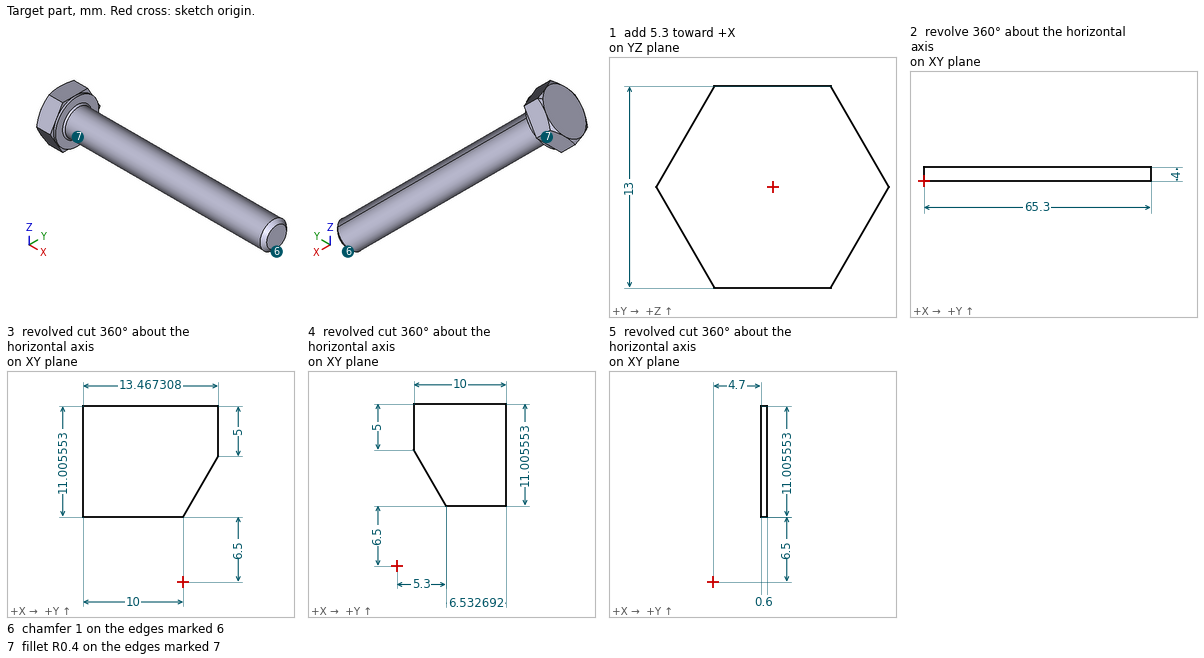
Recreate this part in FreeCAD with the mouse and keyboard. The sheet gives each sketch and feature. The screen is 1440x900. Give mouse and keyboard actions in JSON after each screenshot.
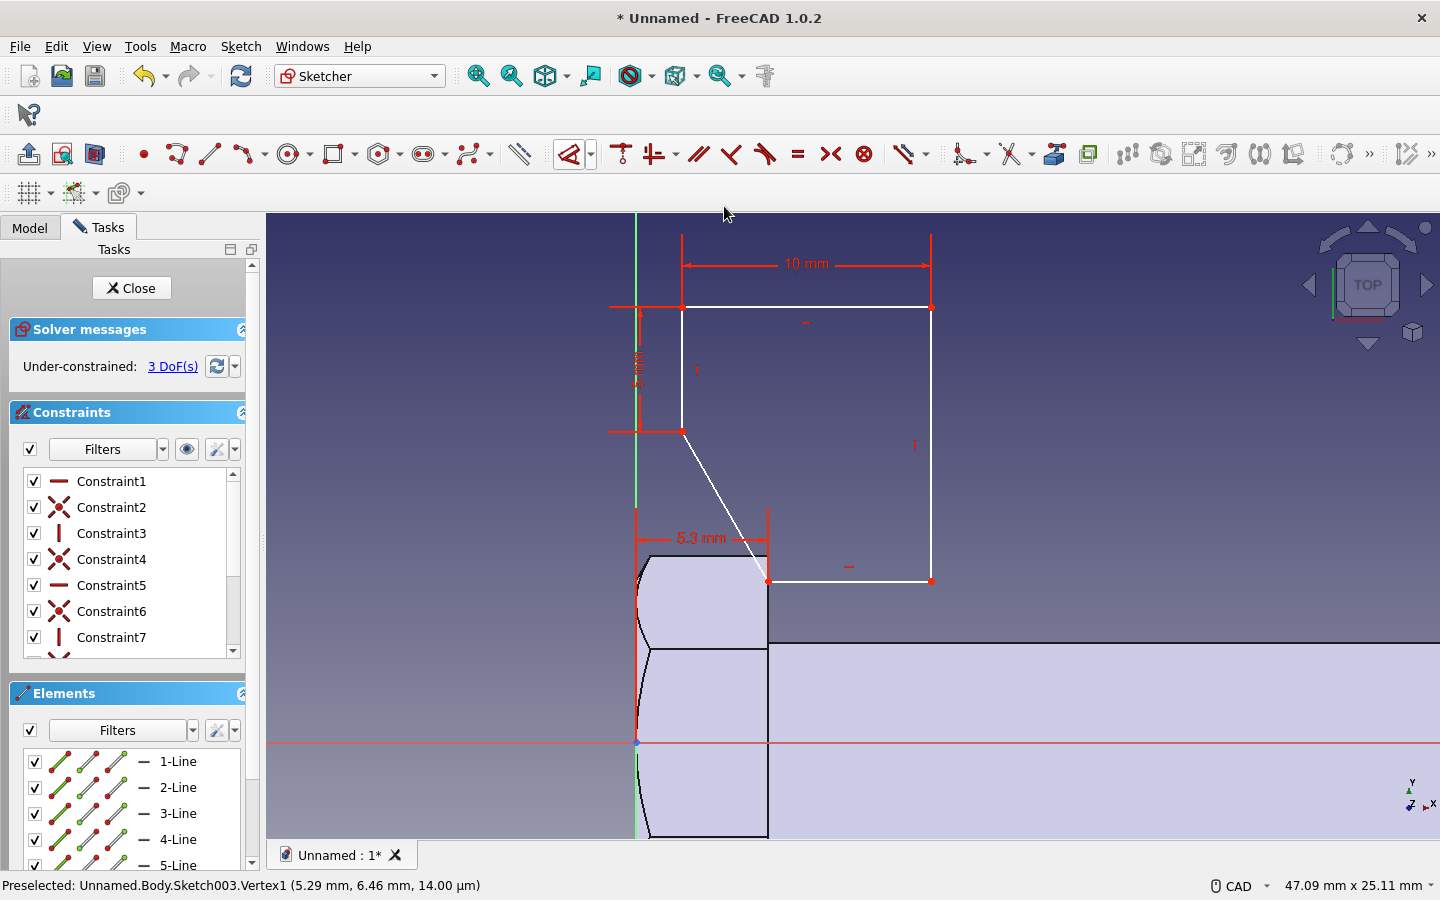
{"action": "left_click", "coordinate": [768, 582]}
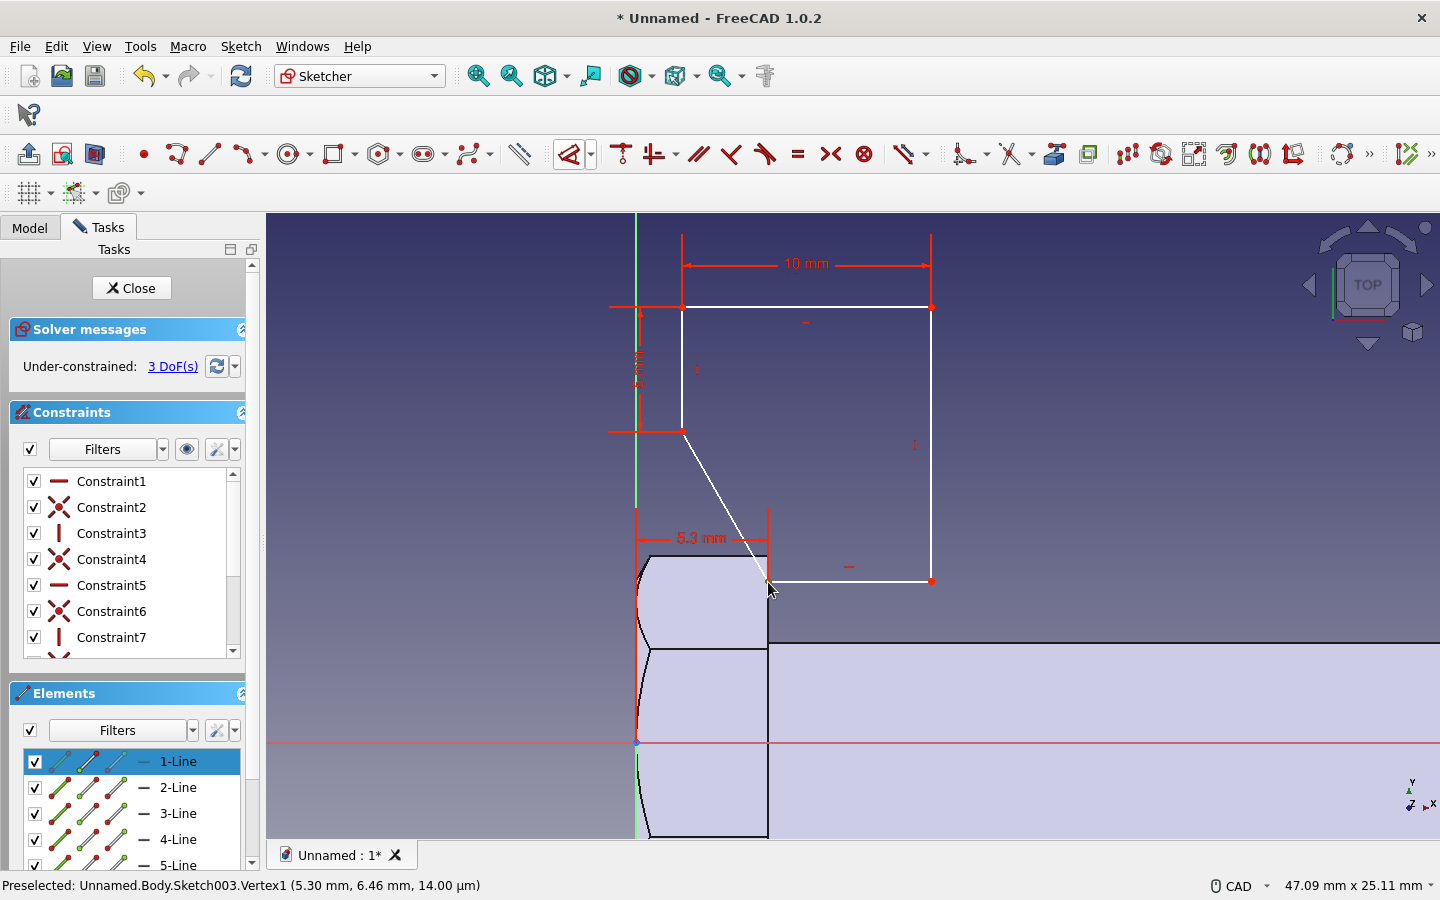
{"action": "key", "text": "i"}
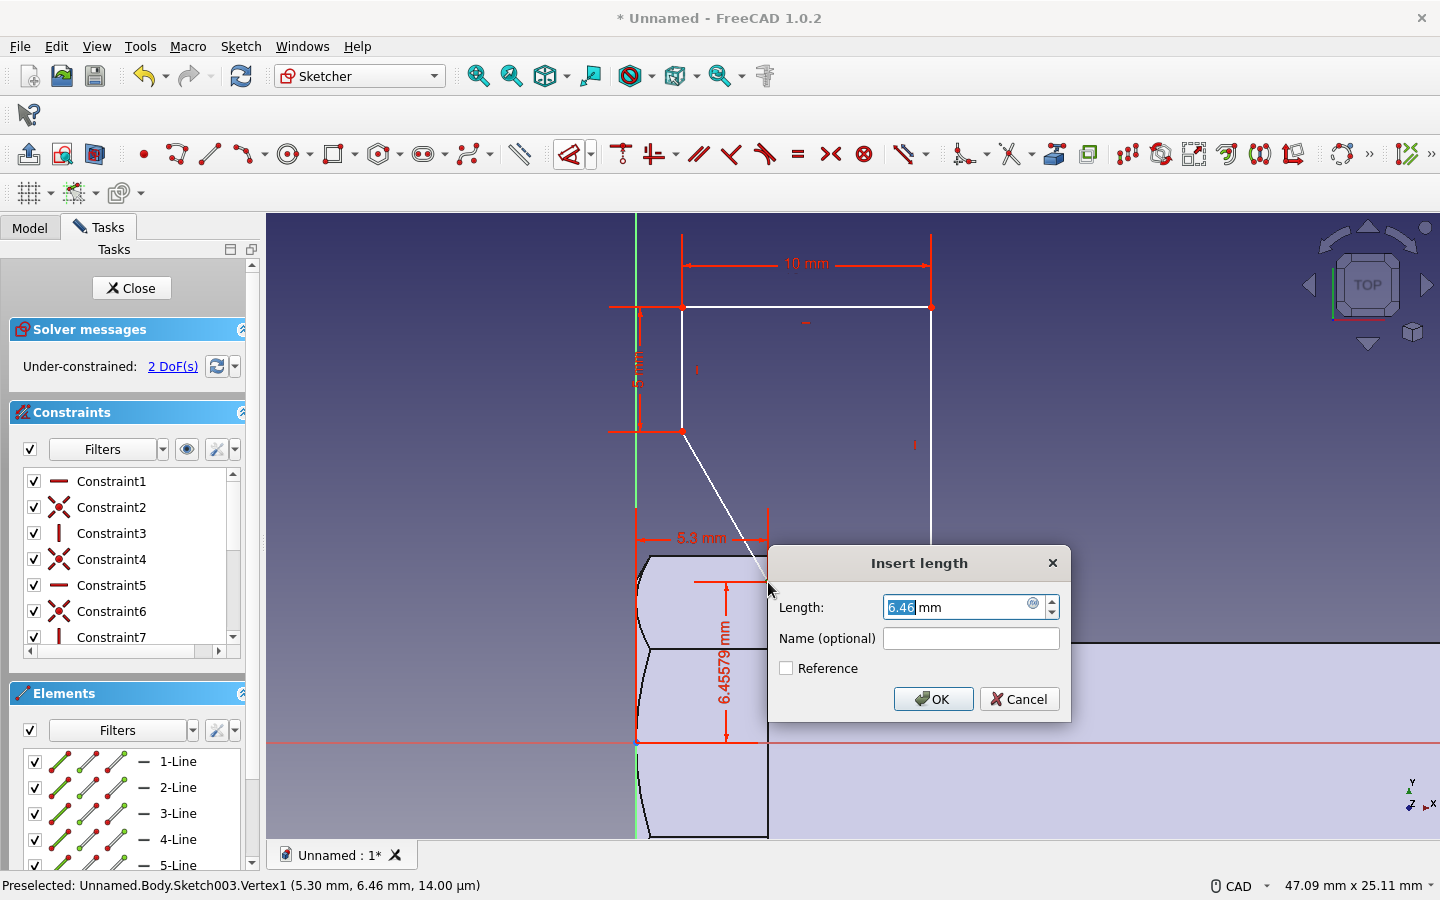
{"action": "type", "text": "6.5"}
{"action": "key", "text": "Return"}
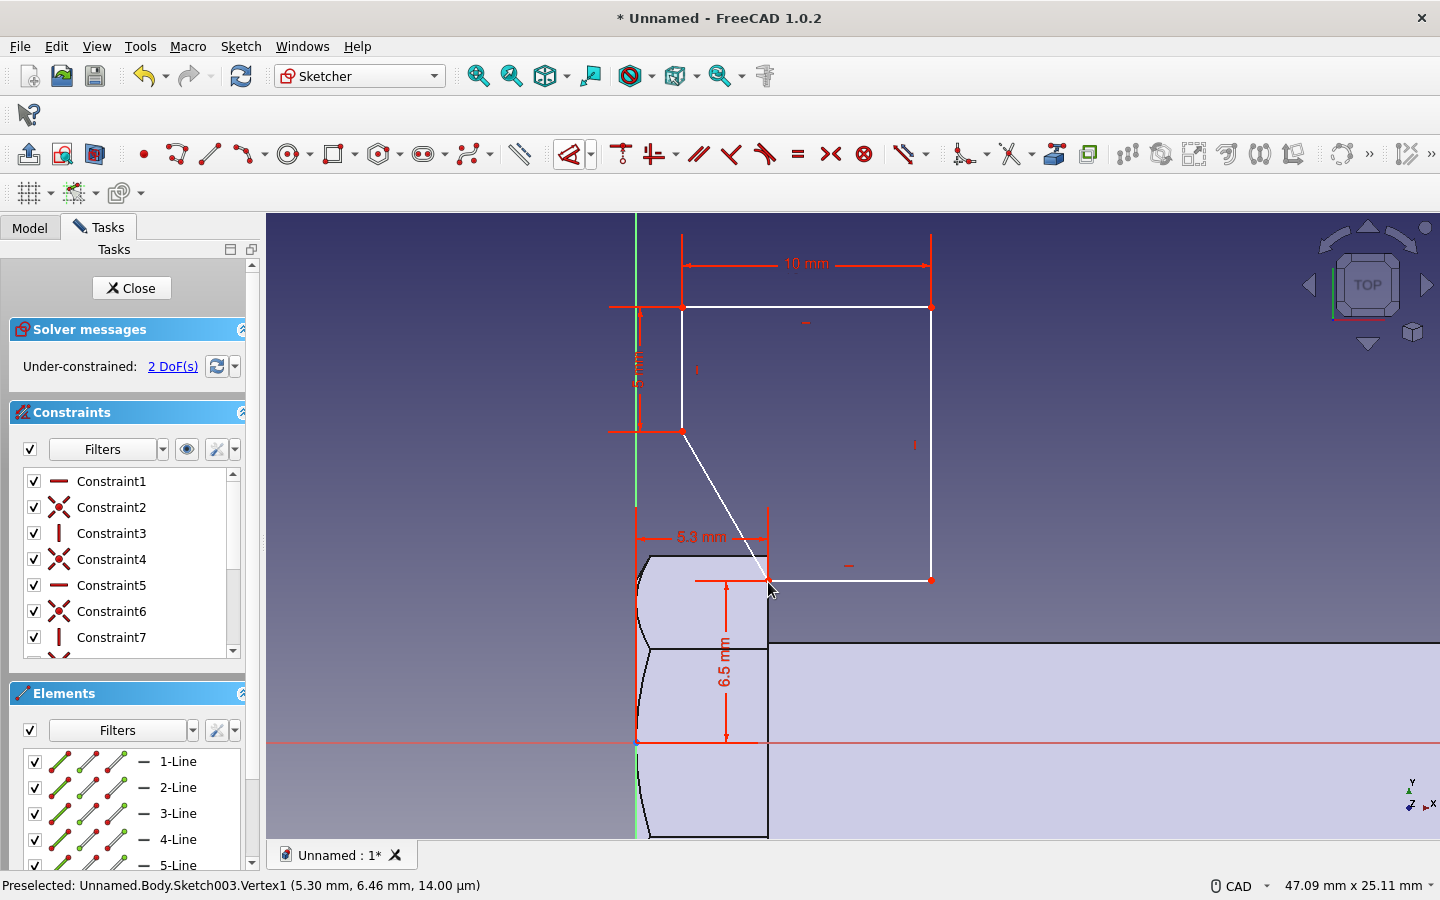
{"action": "left_click", "coordinate": [817, 581]}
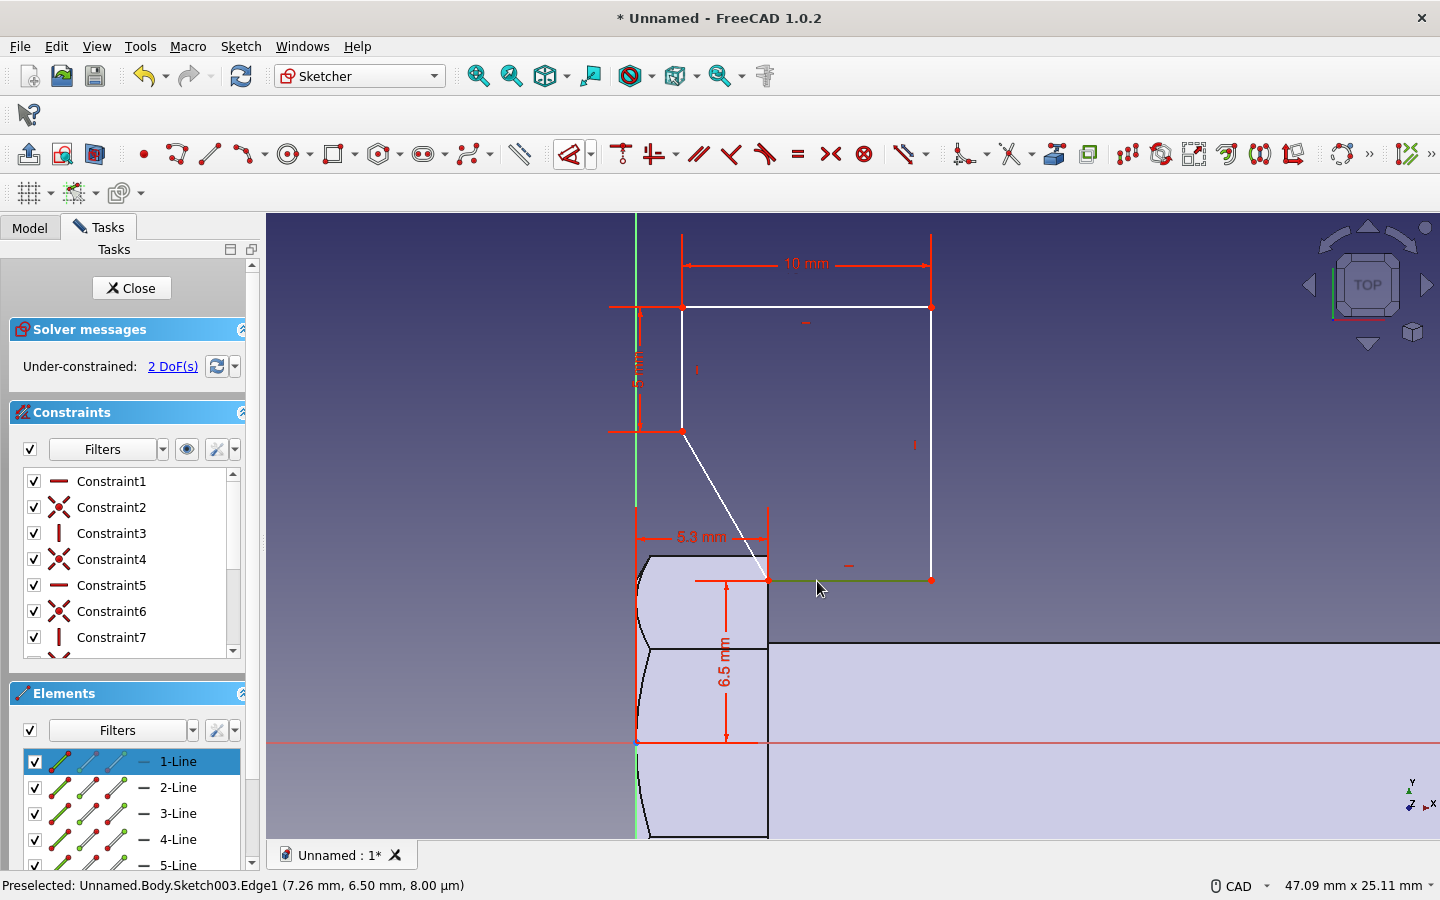
{"action": "key", "text": "l"}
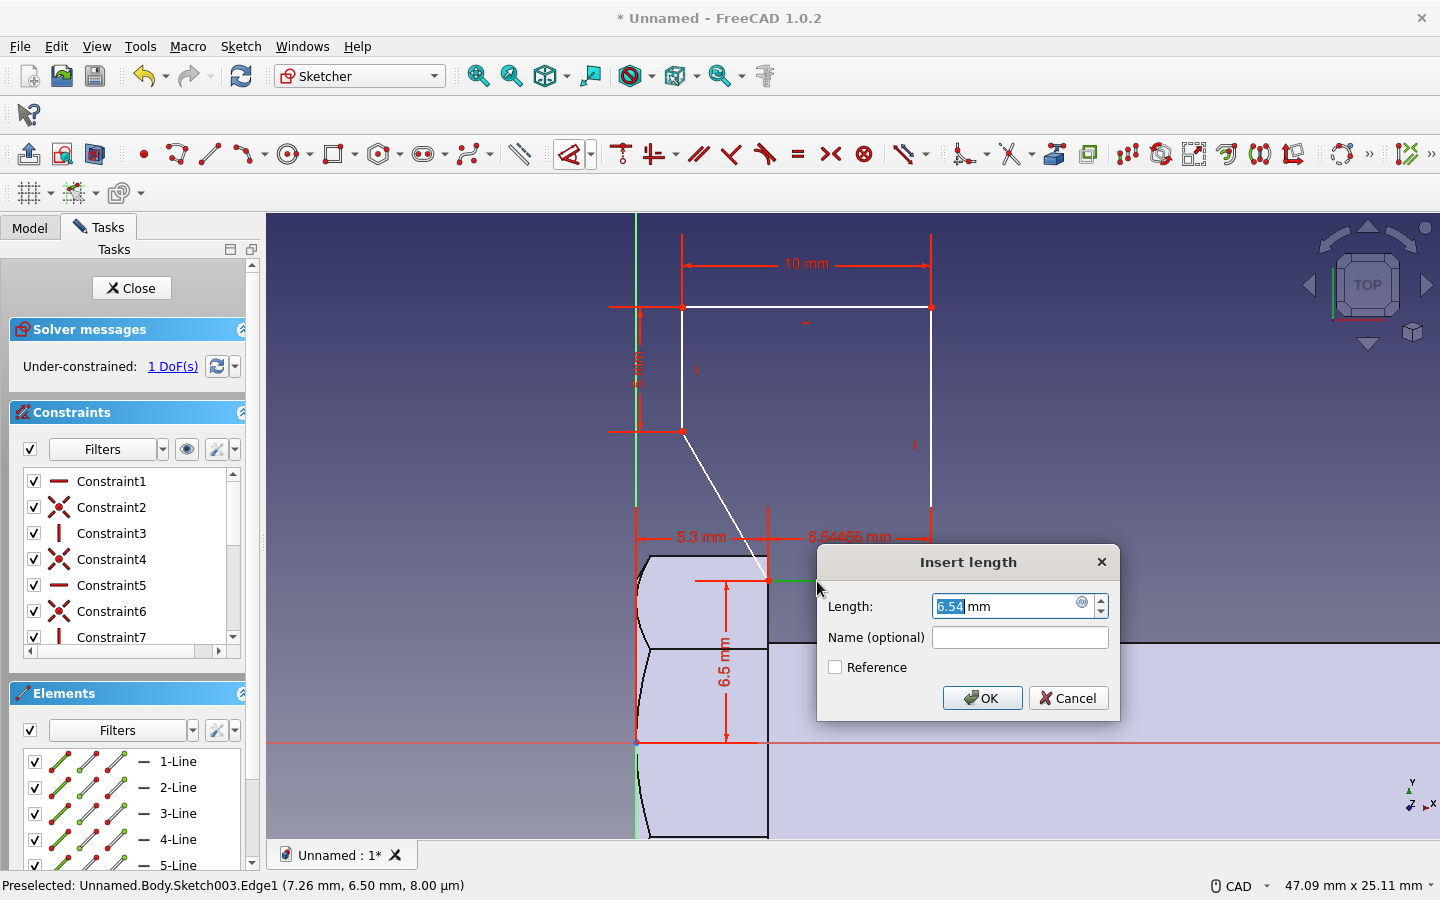
{"action": "type", "text": "6.532692"}
{"action": "key", "text": "Return"}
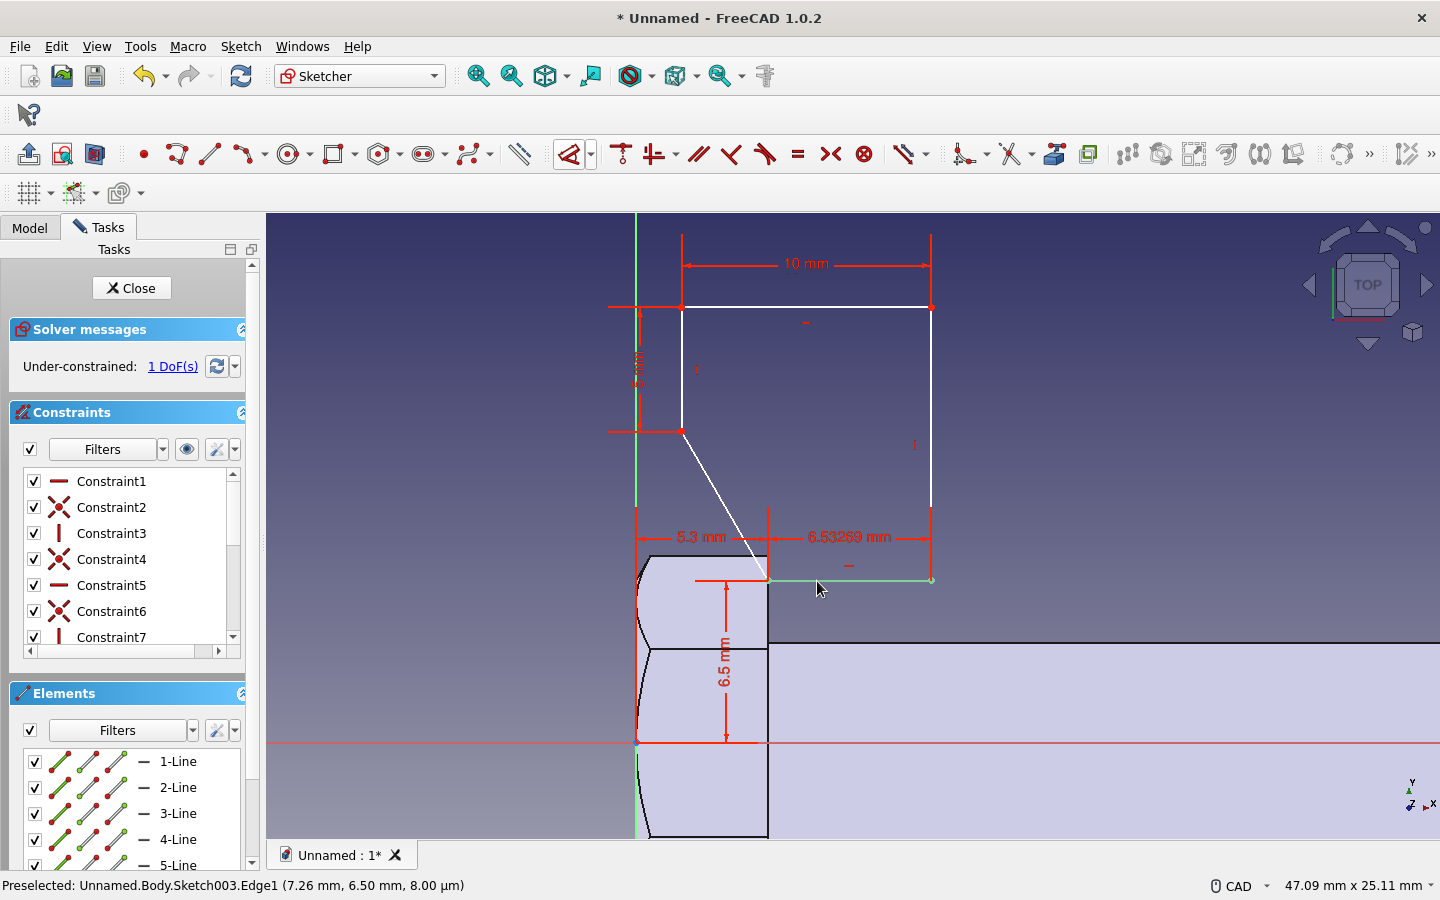
{"action": "left_click", "coordinate": [931, 499]}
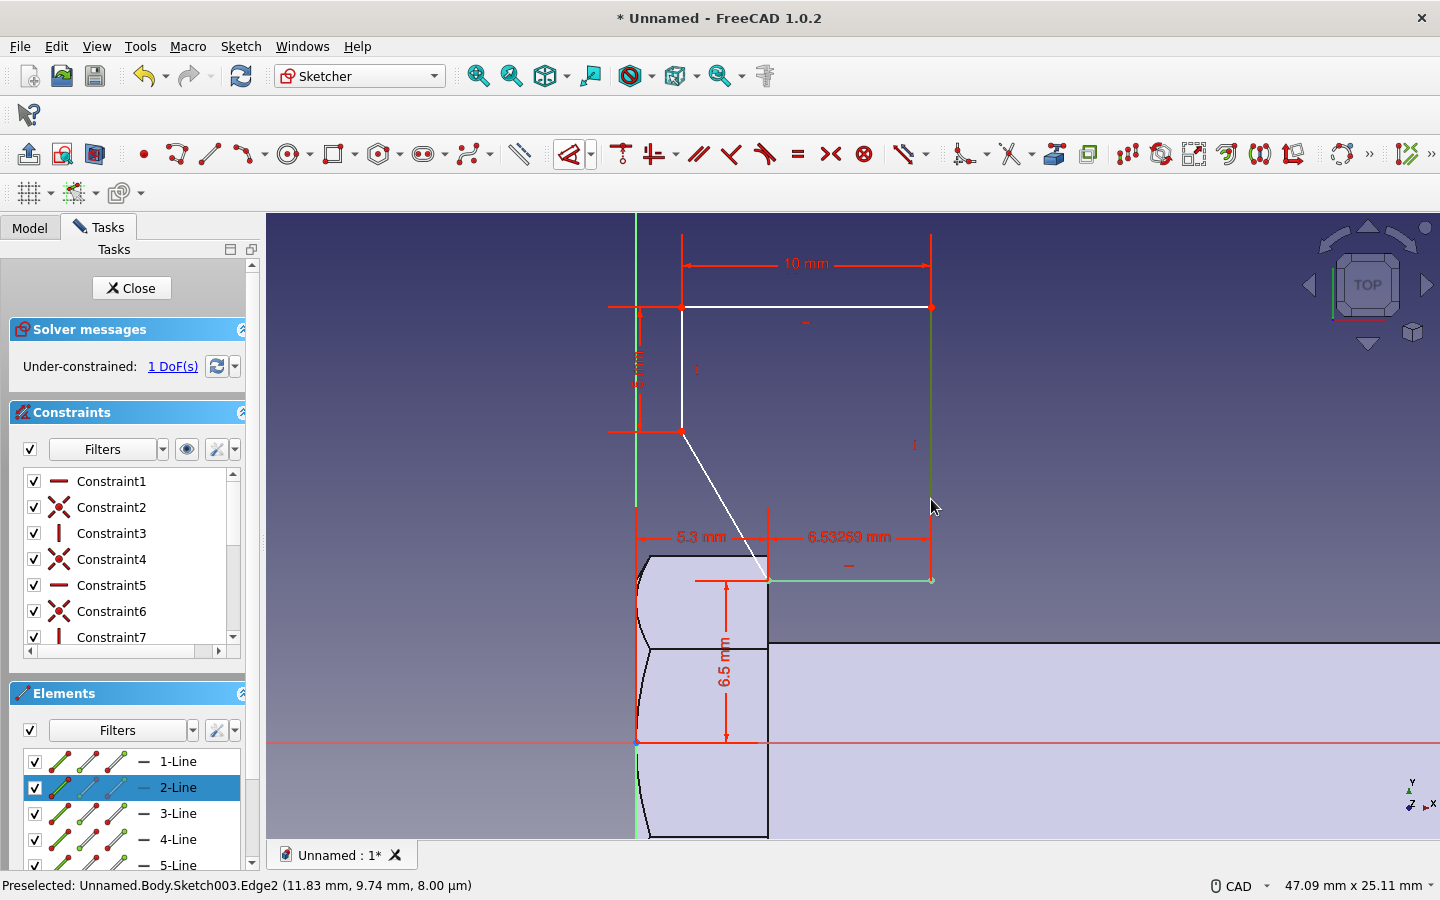
{"action": "left_click", "coordinate": [590, 154]}